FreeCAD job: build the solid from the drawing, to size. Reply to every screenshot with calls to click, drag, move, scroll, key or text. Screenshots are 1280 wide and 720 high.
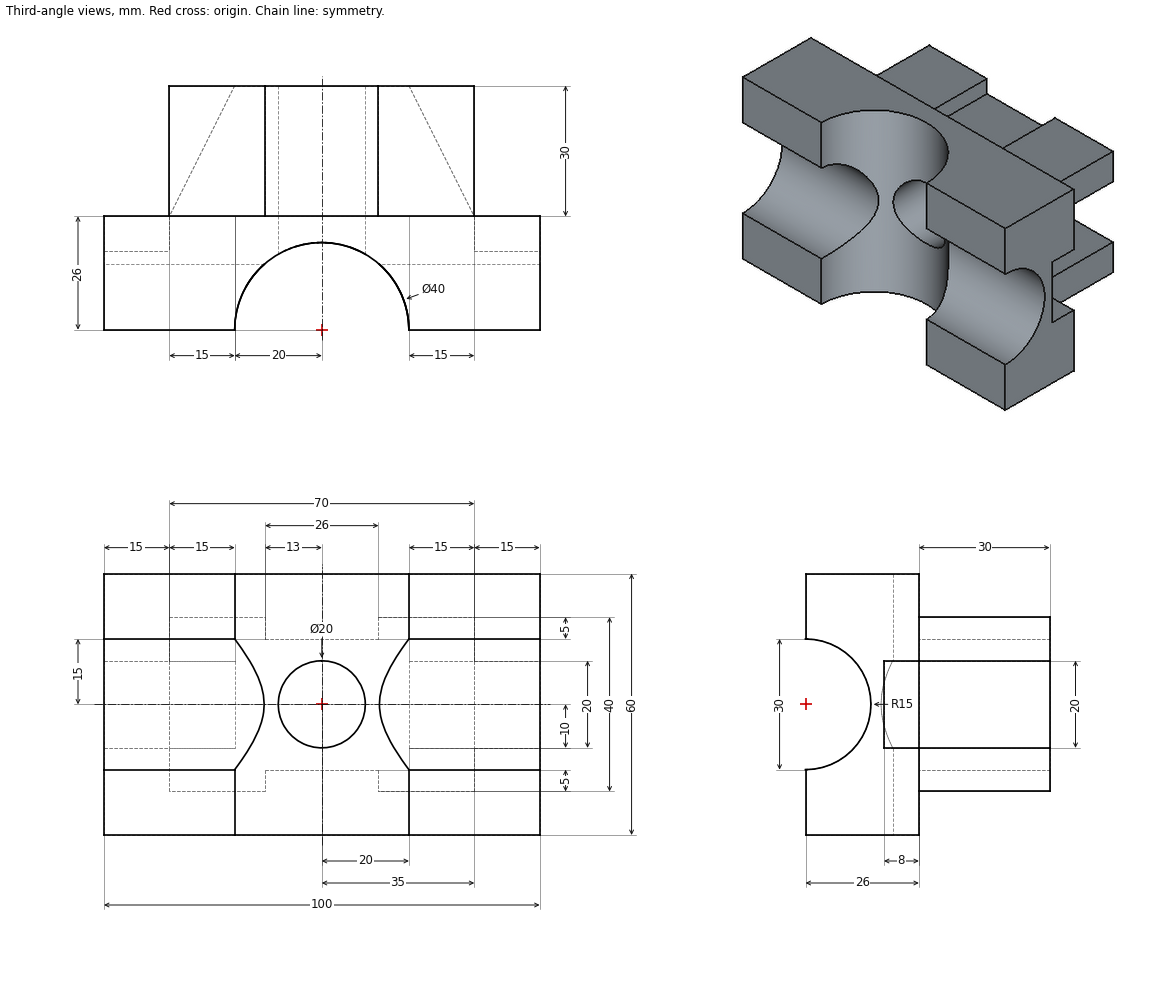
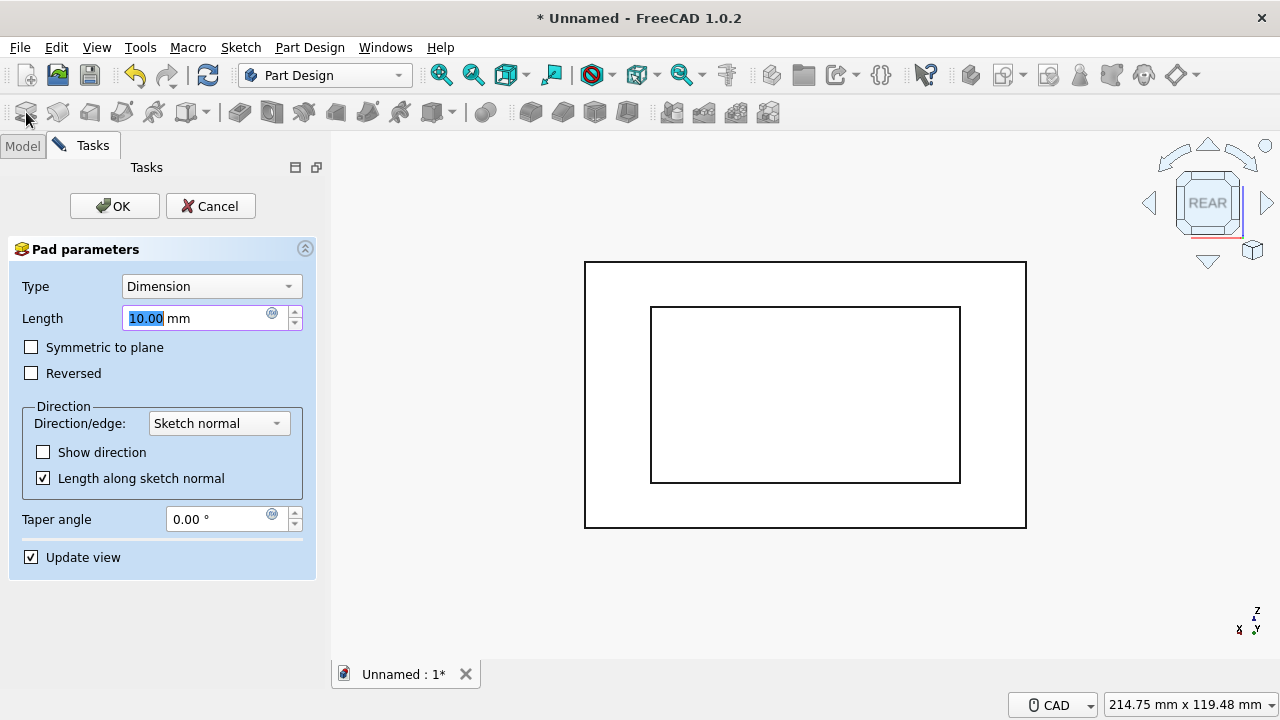
text(30)
key(Tab)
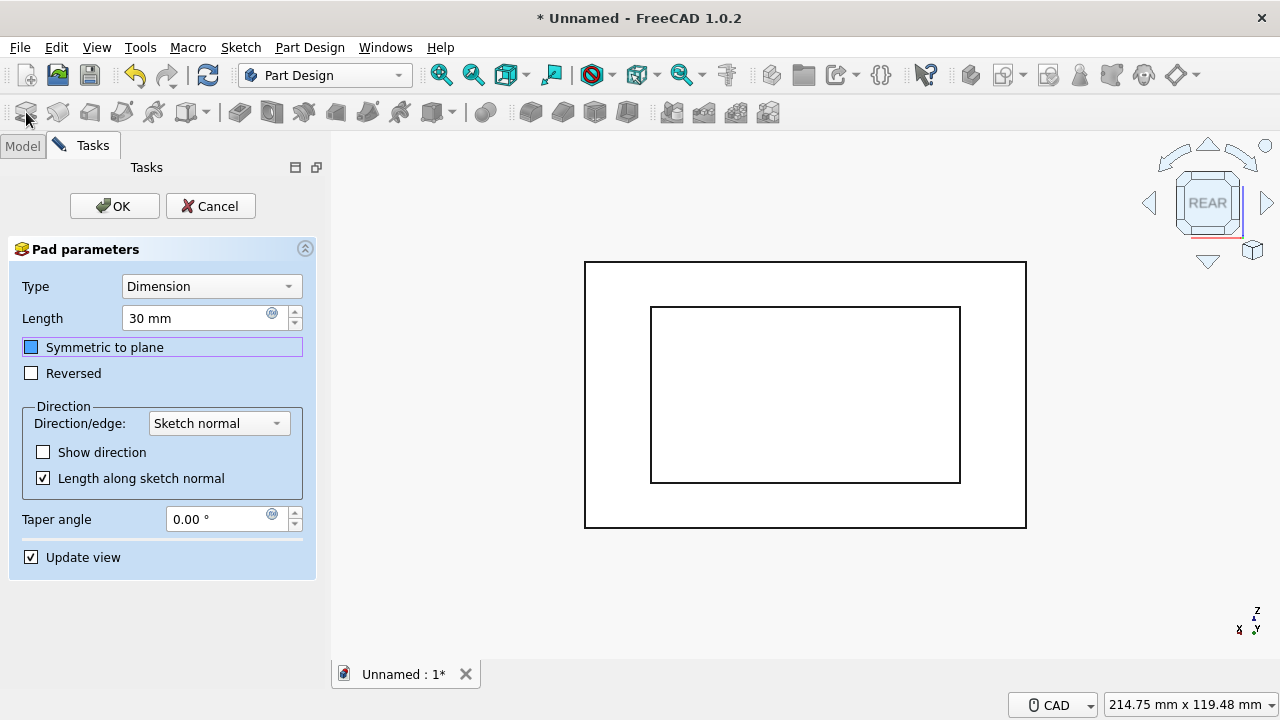
click(115, 206)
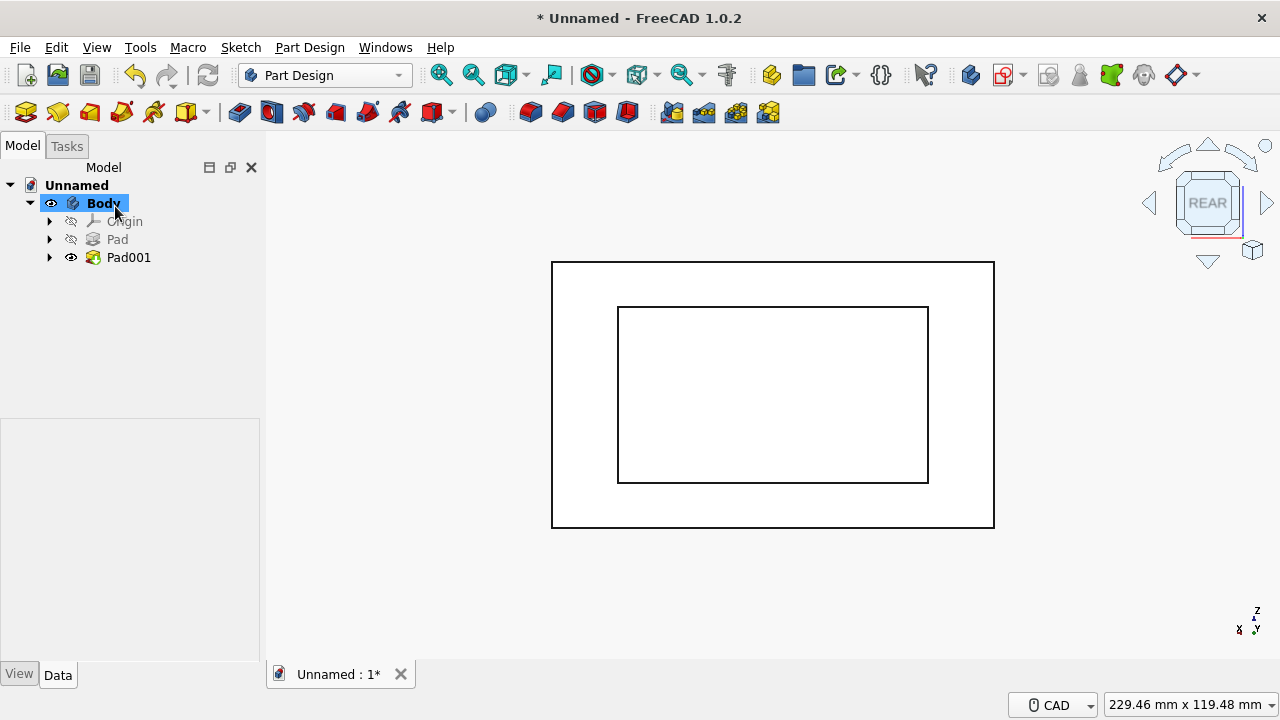
click(729, 394)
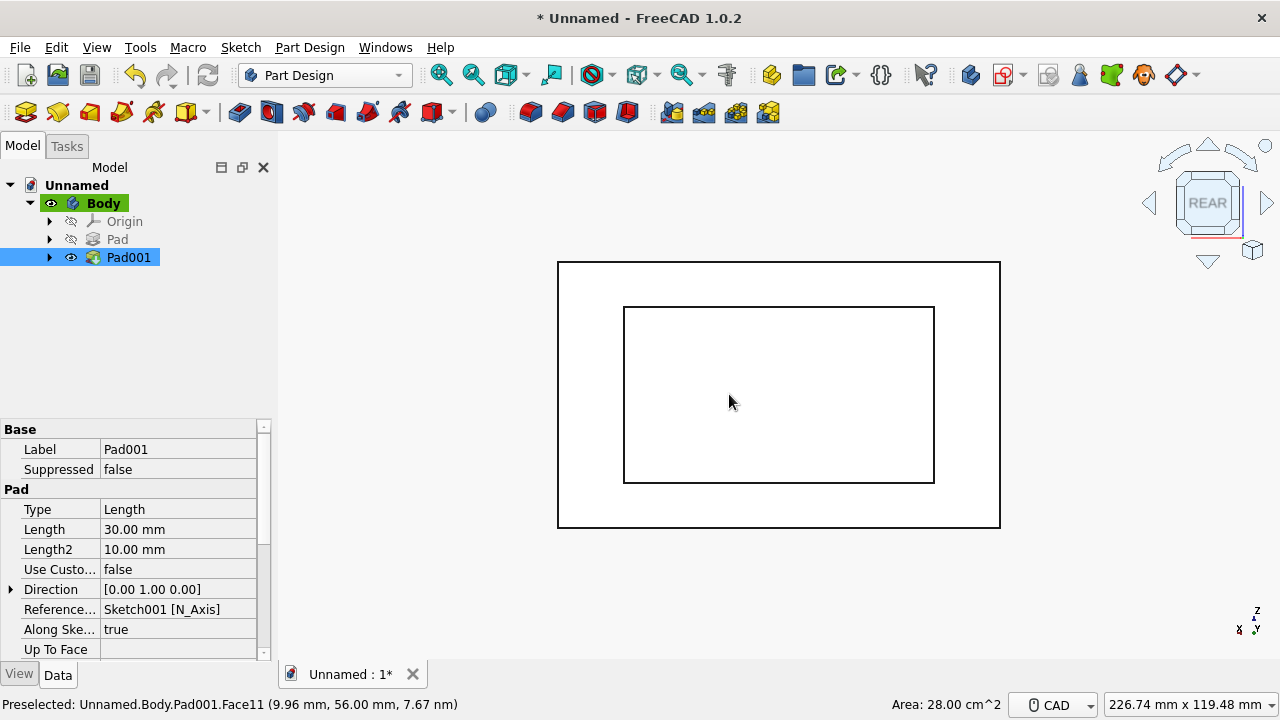
click(1004, 76)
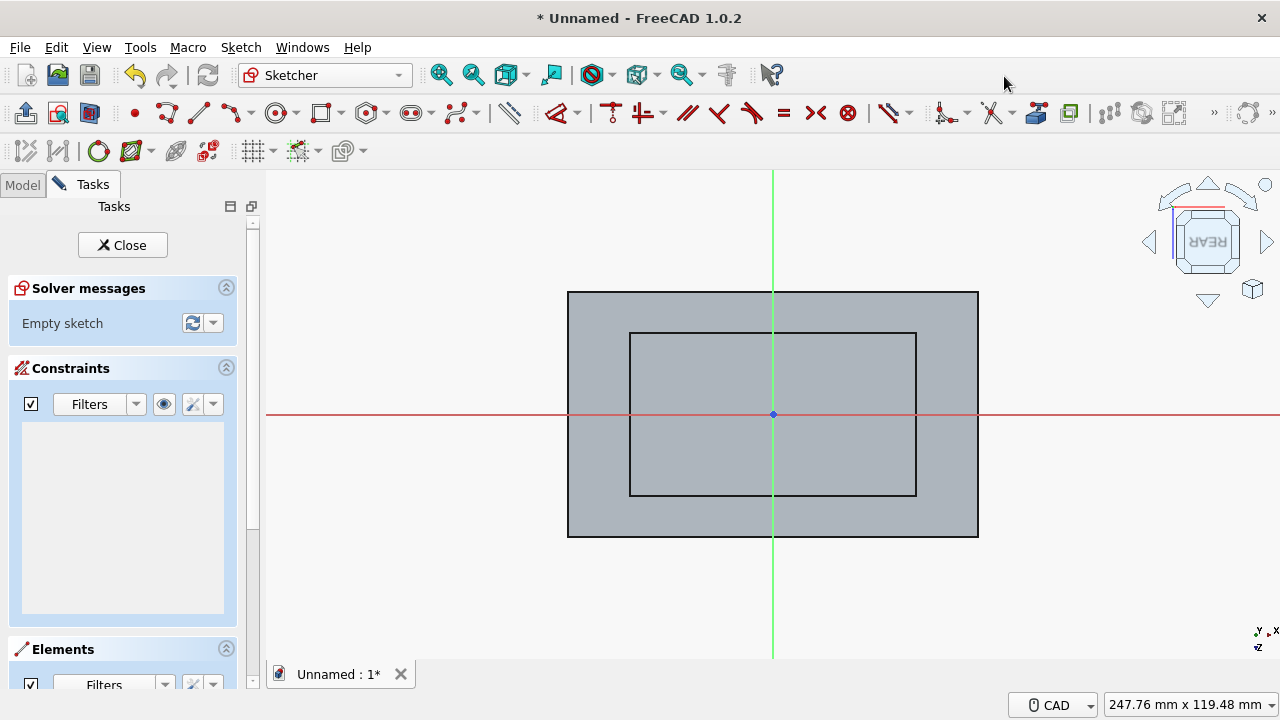
scroll(856, 414, up, 3)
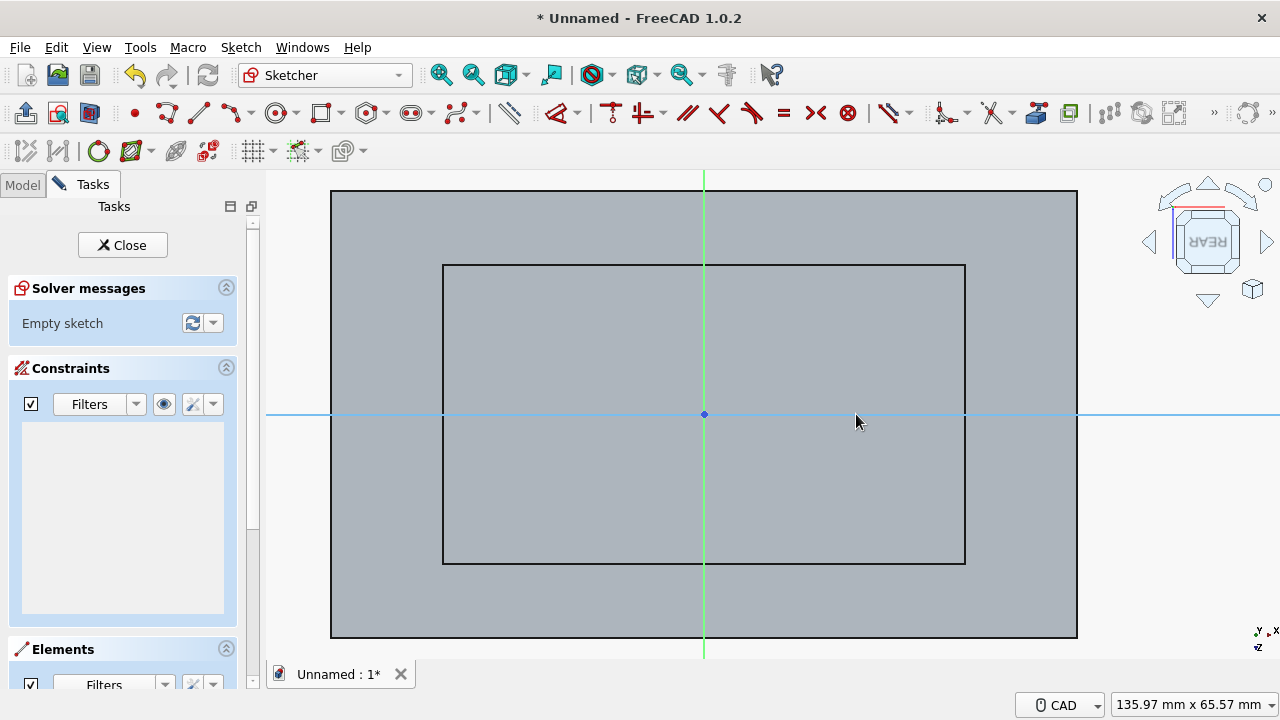
key(g)
key(r)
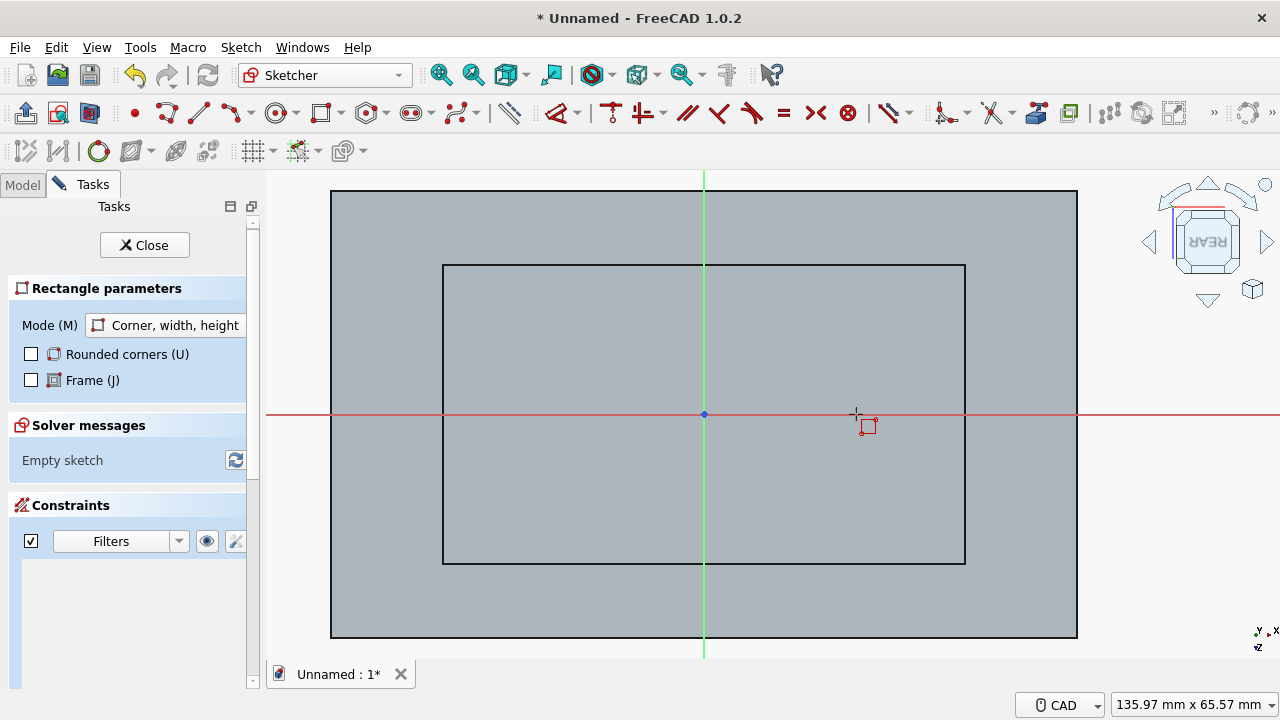
click(853, 340)
move(965, 489)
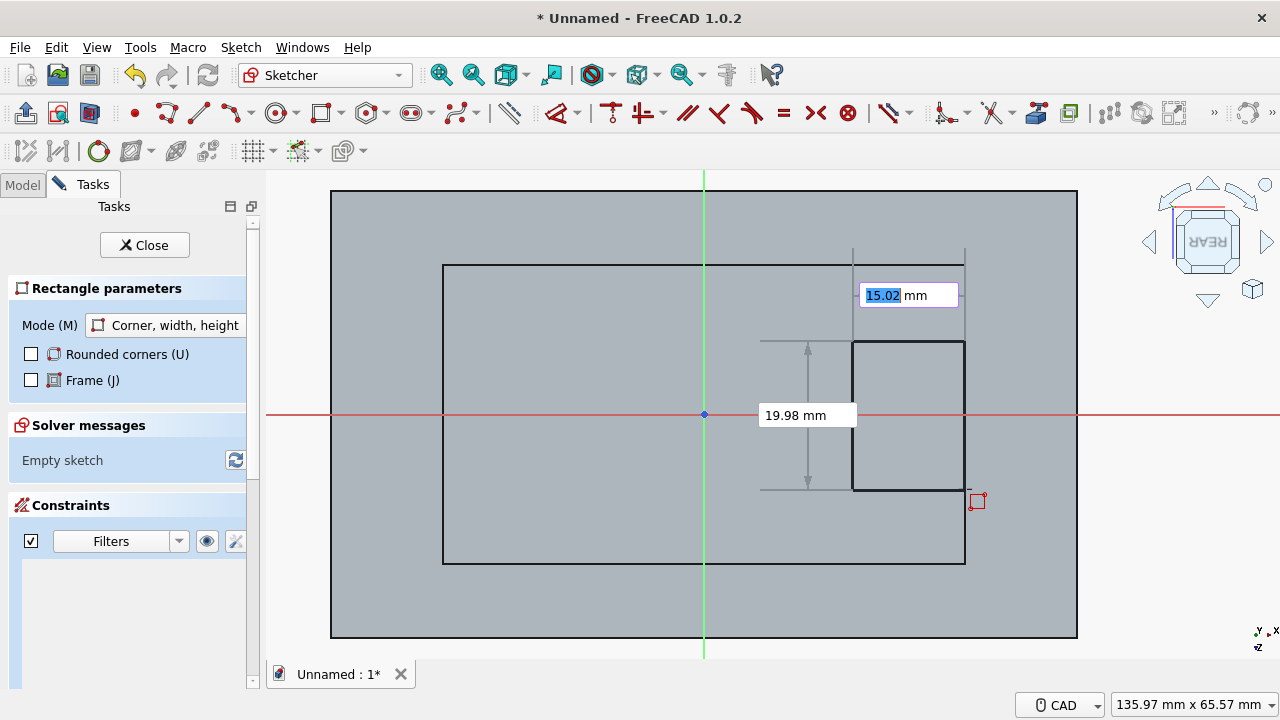
text(15)
key(Tab)
text(20)
key(Return)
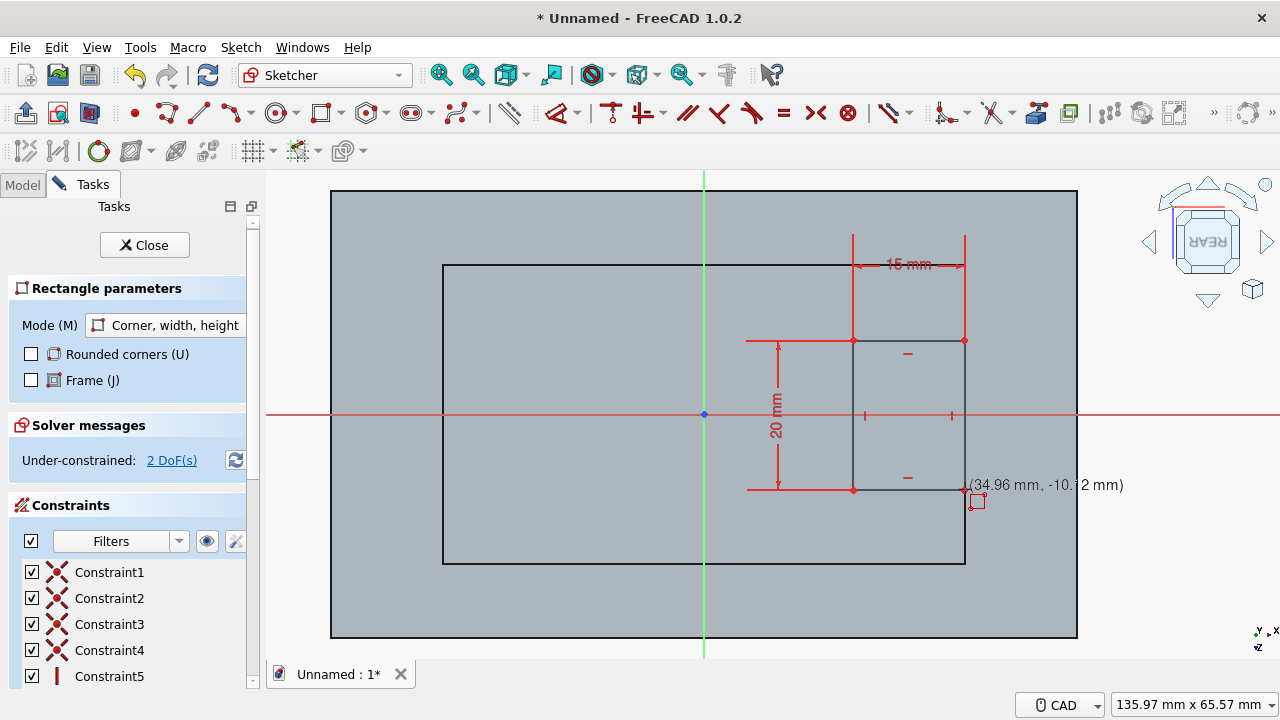
click(607, 526)
move(801, 564)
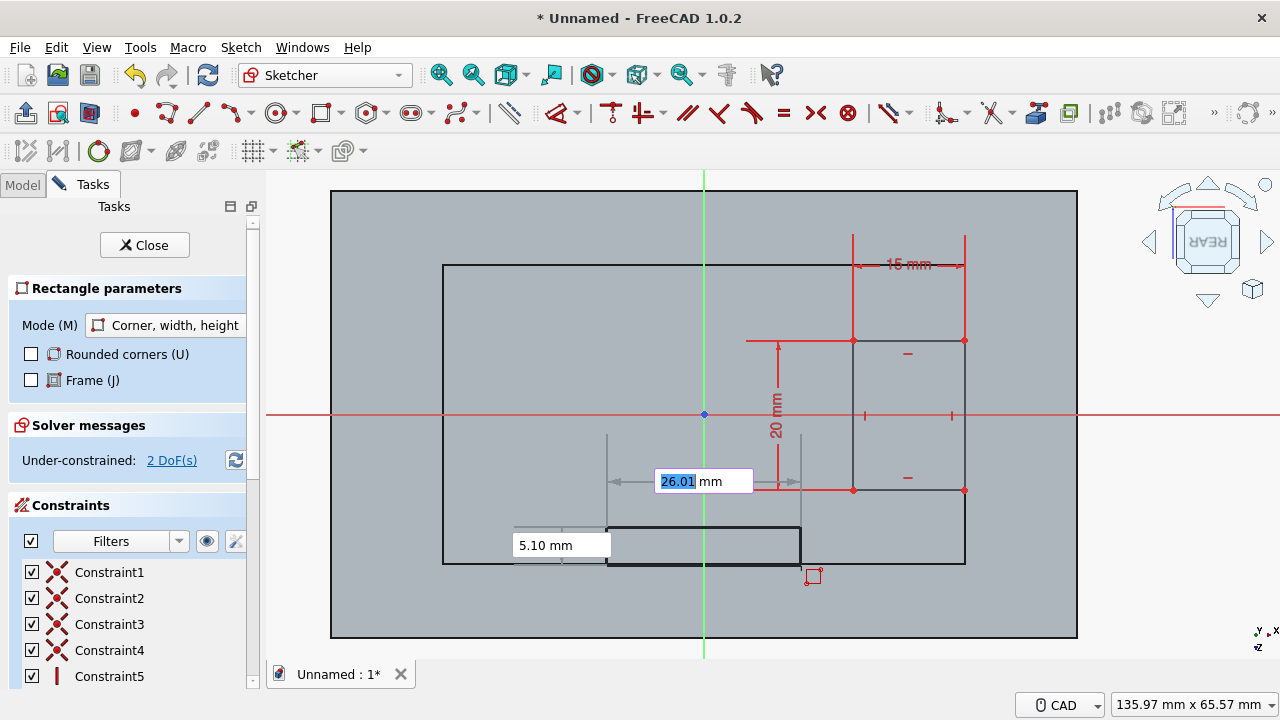
text(26)
key(Tab)
text(5)
key(Return)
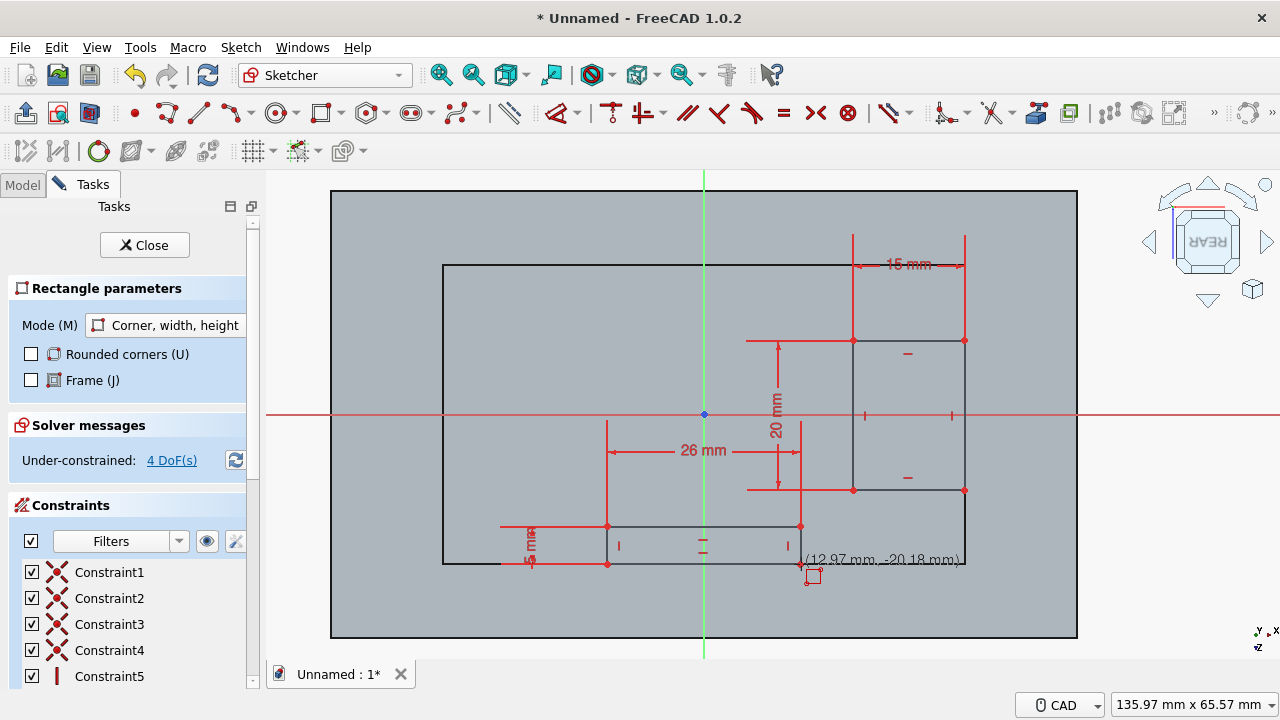
click(443, 340)
move(555, 489)